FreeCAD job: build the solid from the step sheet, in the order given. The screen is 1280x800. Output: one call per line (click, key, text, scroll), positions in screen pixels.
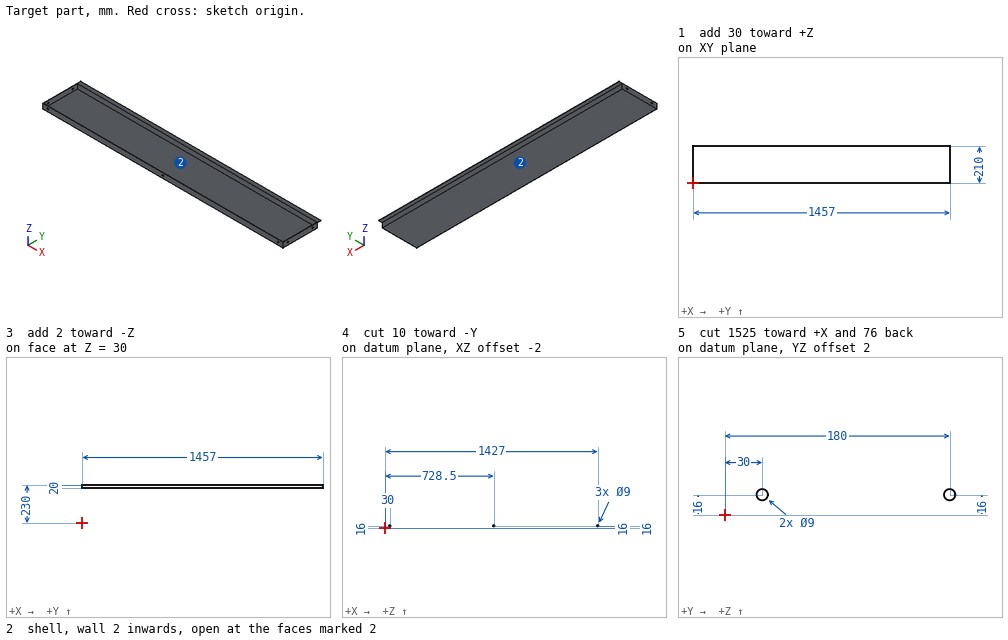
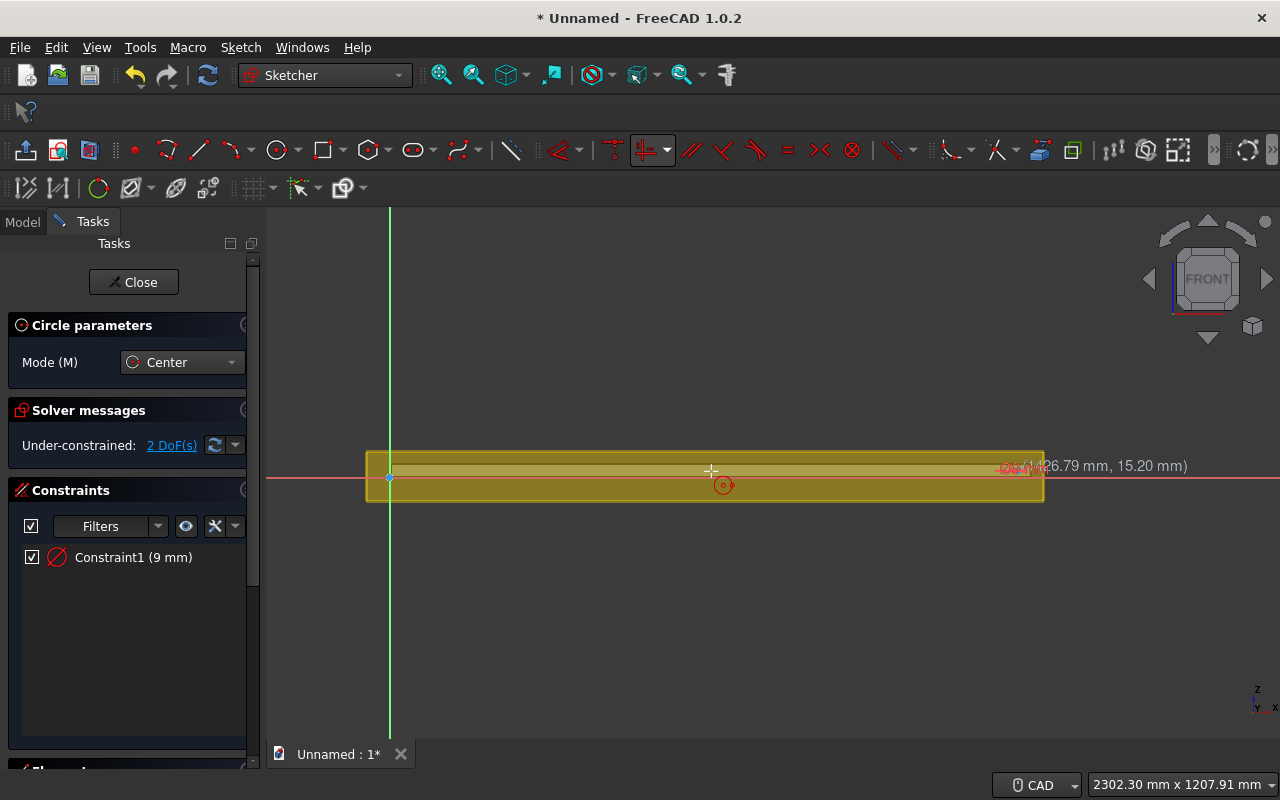
scroll(711, 471, up, 5)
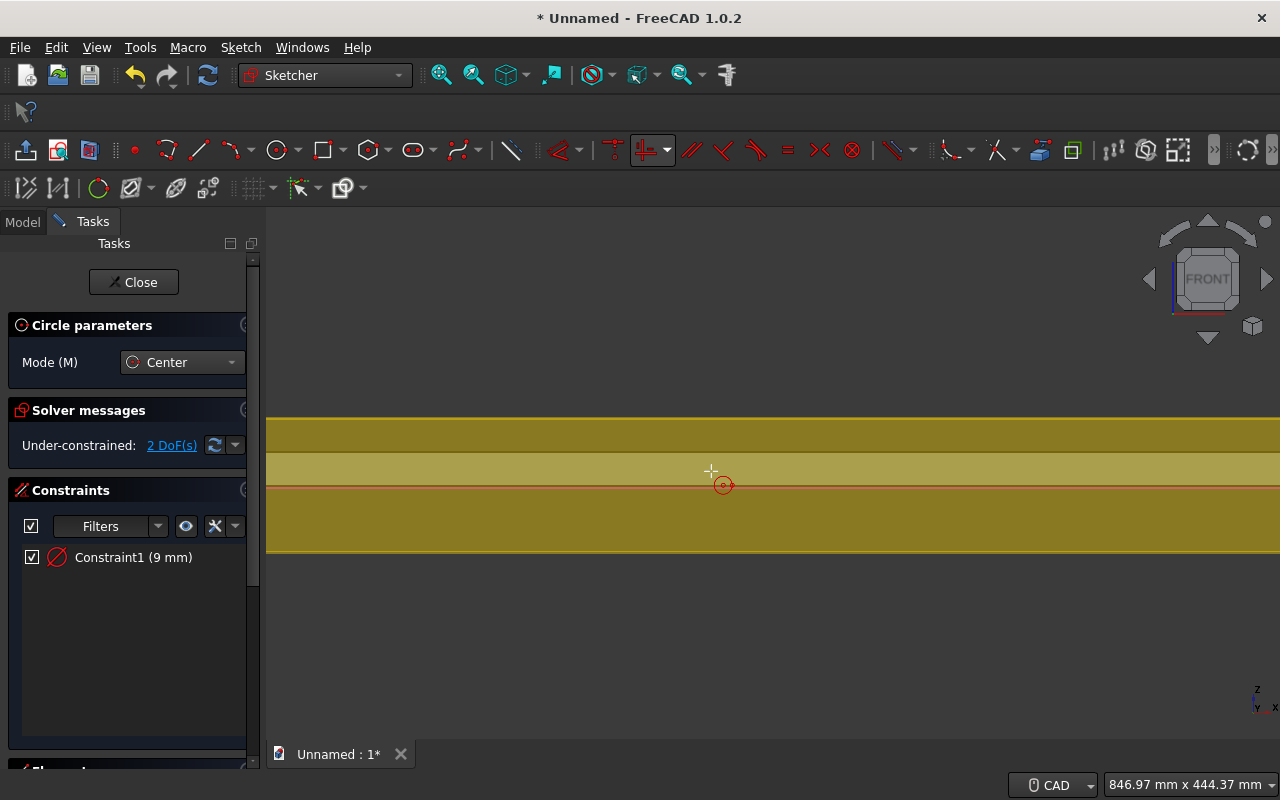
click(709, 469)
move(713, 465)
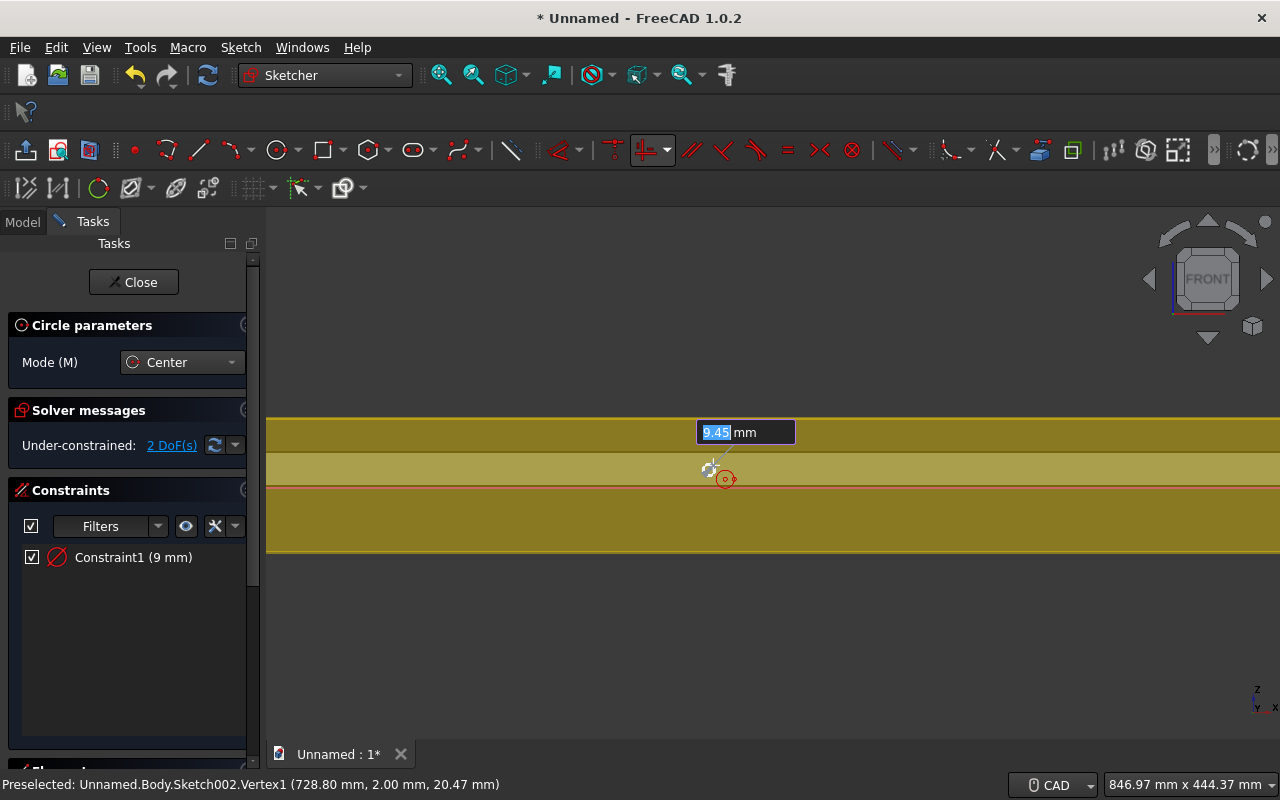
text(9)
key(Return)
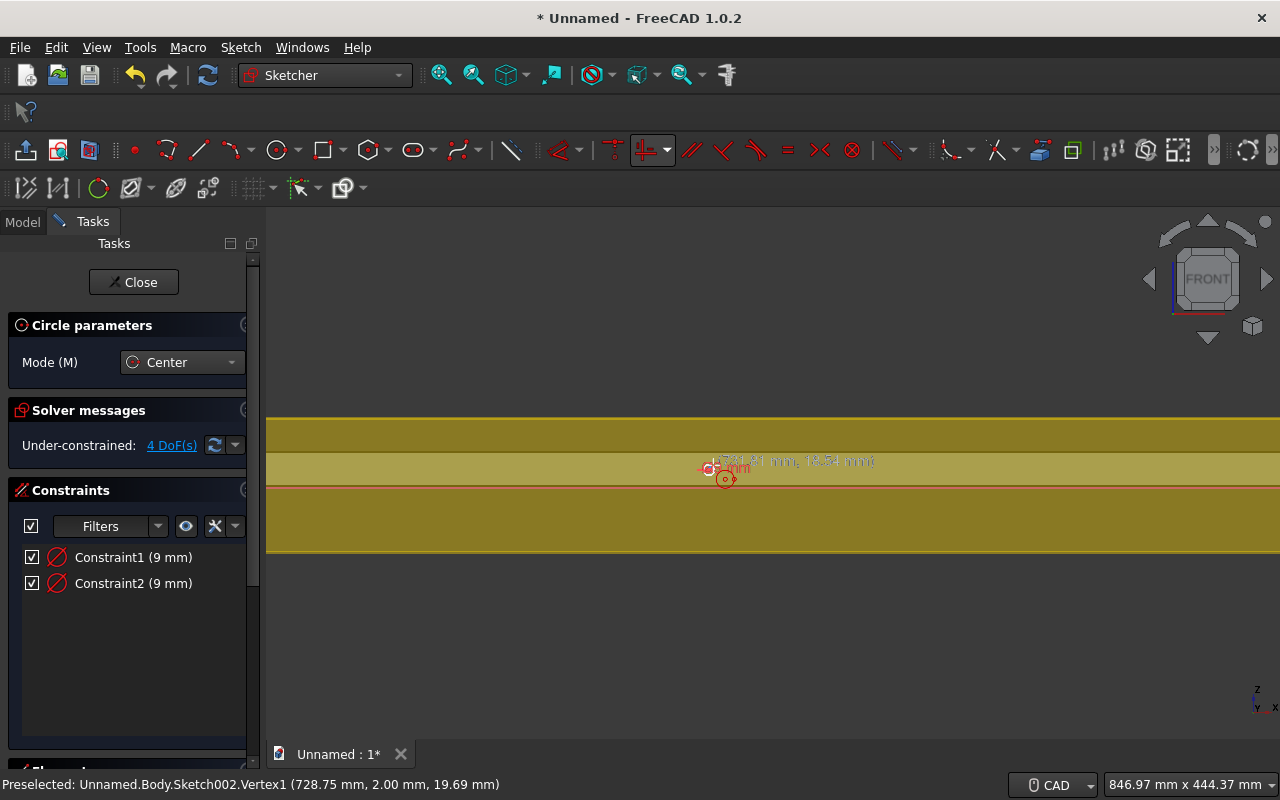
scroll(711, 471, down, 5)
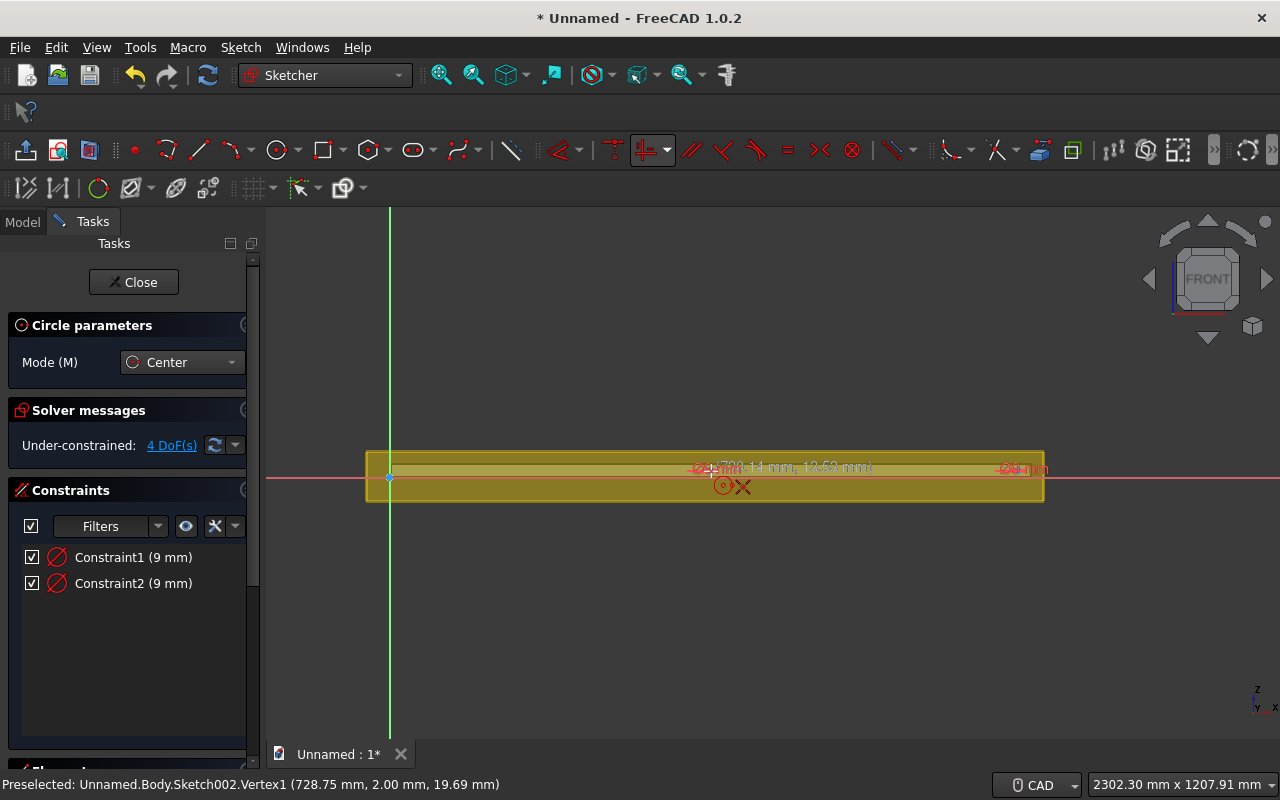
scroll(403, 471, up, 13)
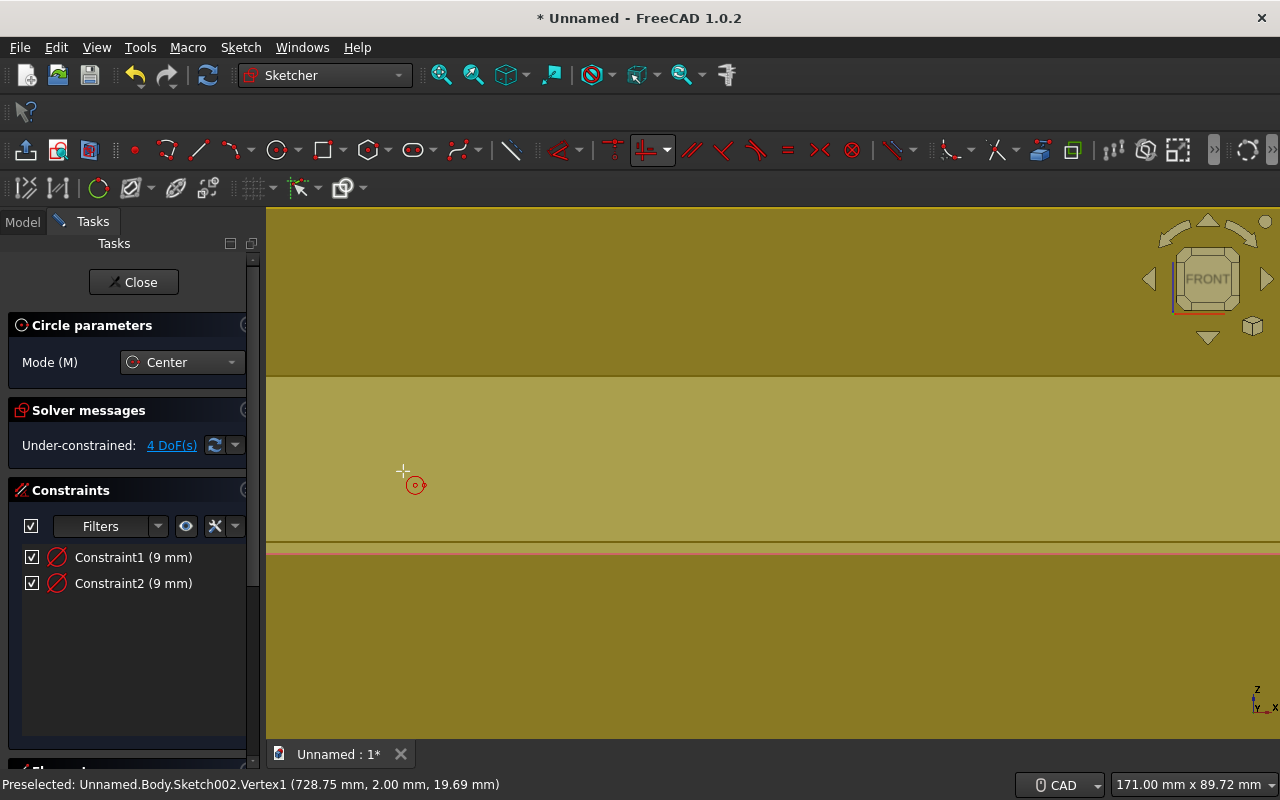
scroll(403, 471, down, 13)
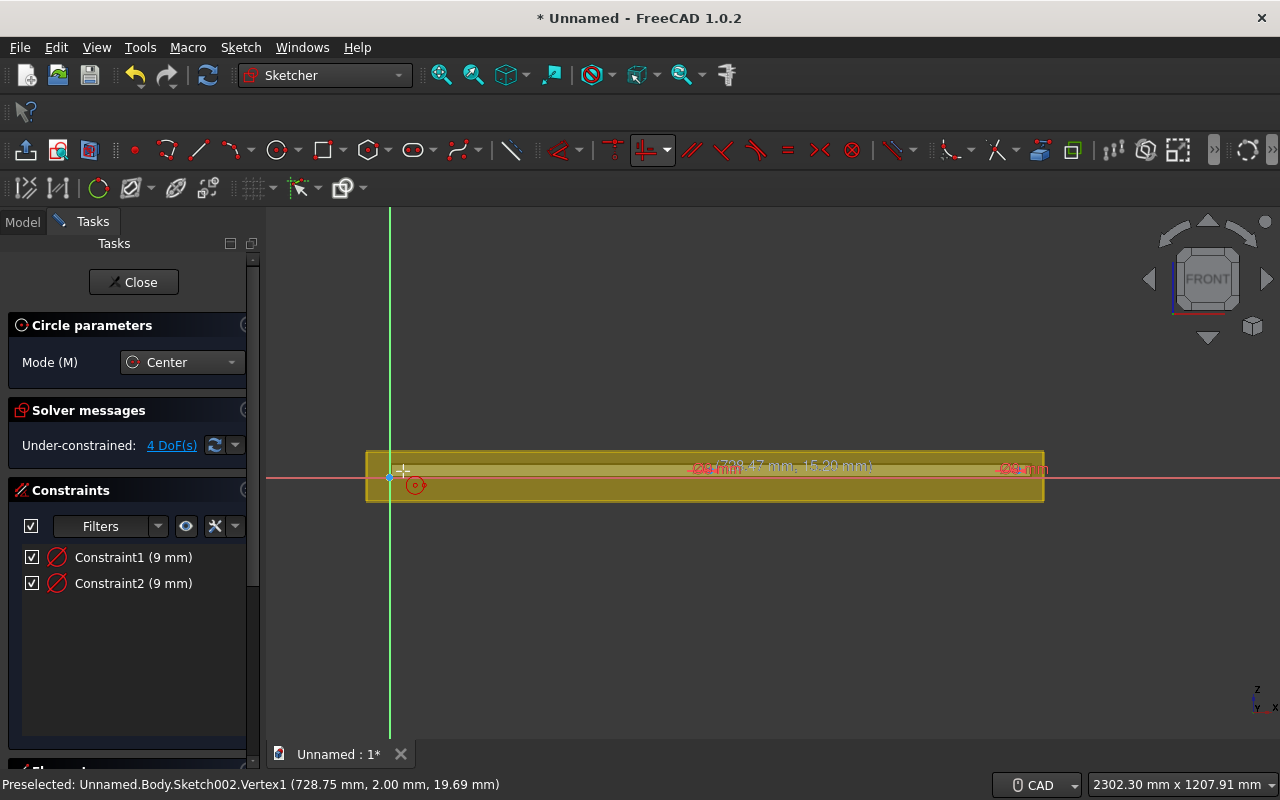
scroll(403, 471, up, 5)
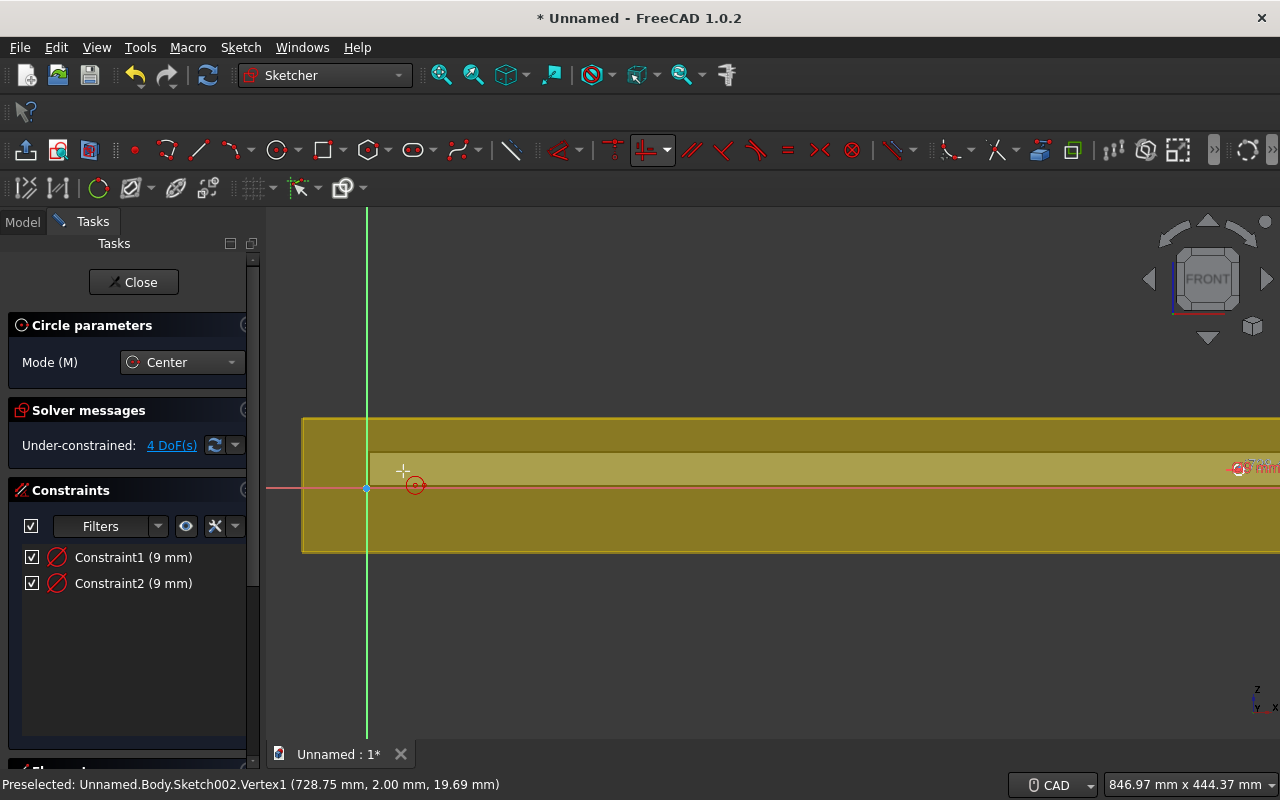
click(403, 469)
move(406, 465)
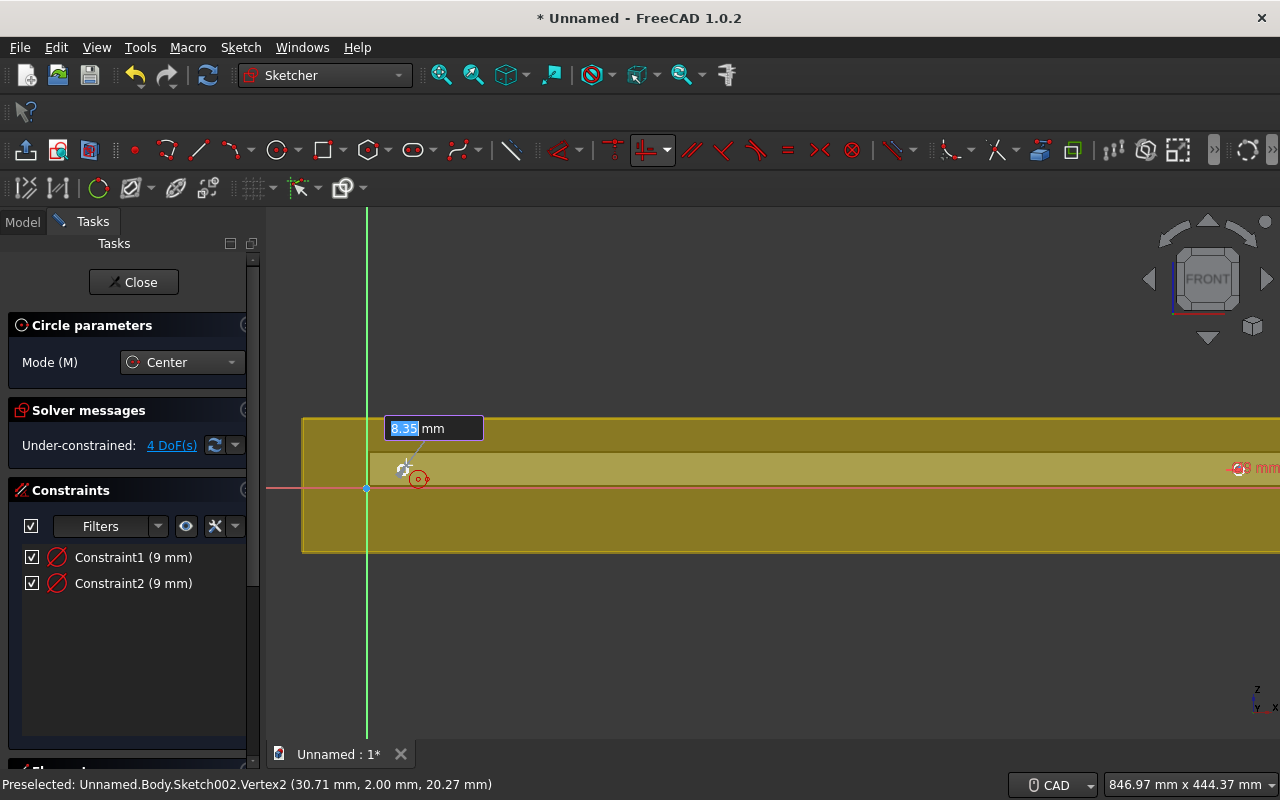
text(9)
key(Return)
key(Escape)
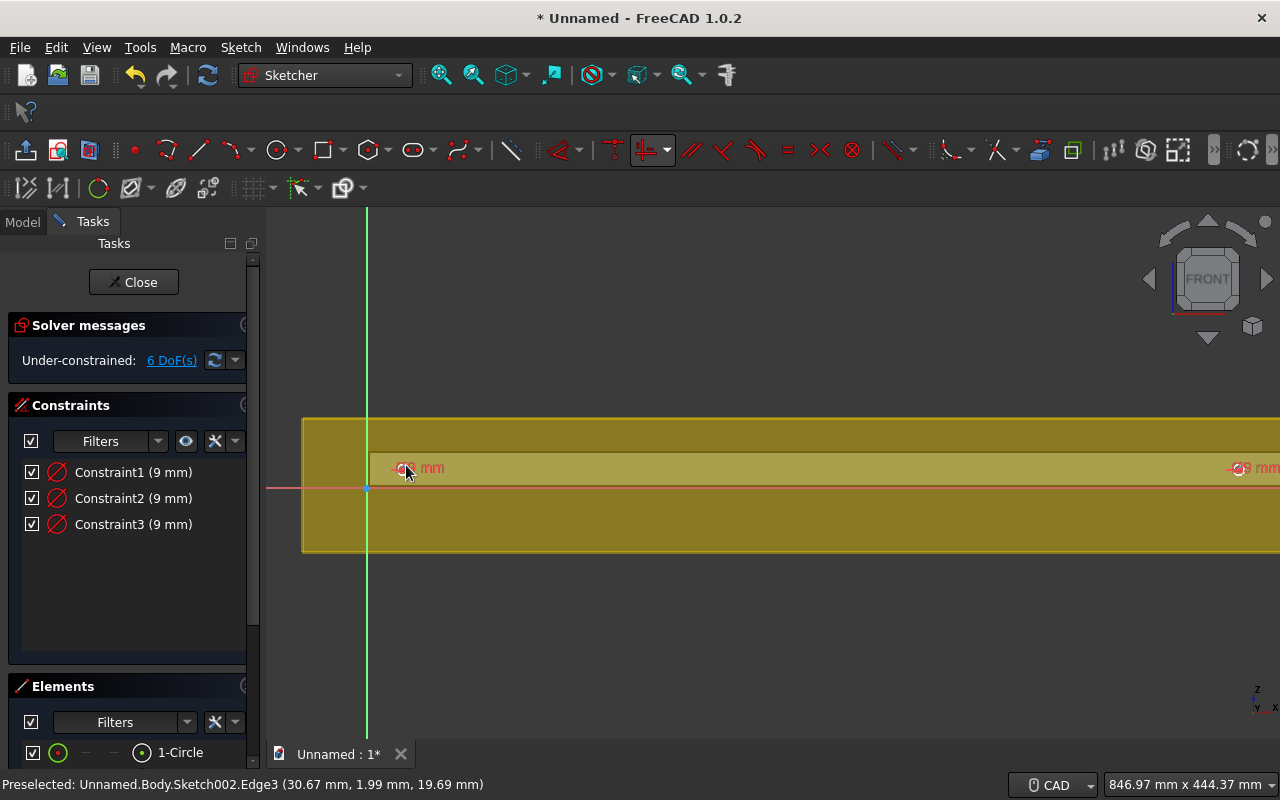
click(558, 150)